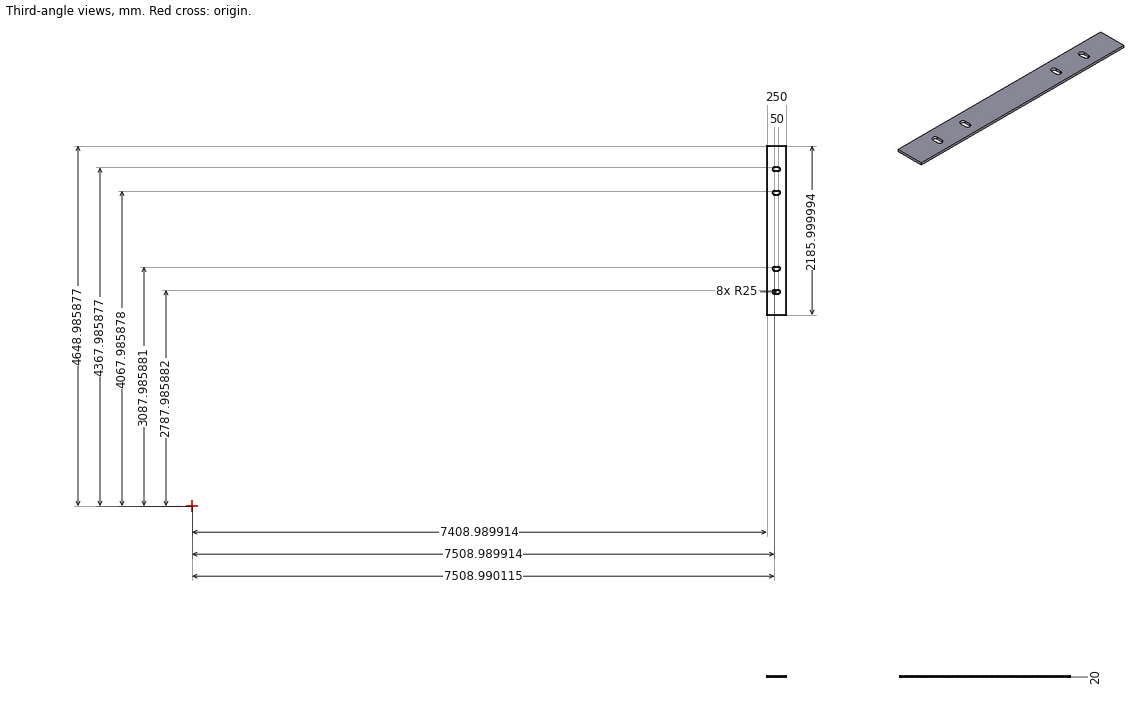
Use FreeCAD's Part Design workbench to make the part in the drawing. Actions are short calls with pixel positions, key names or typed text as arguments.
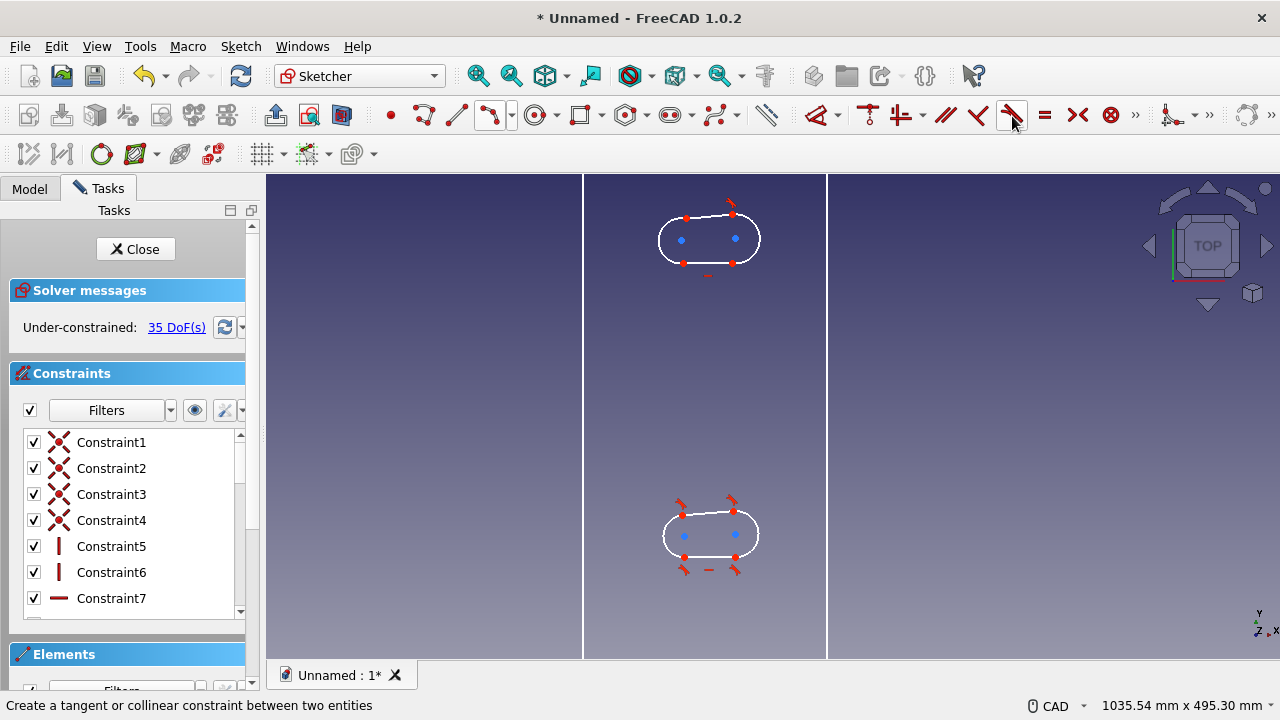
click(700, 218)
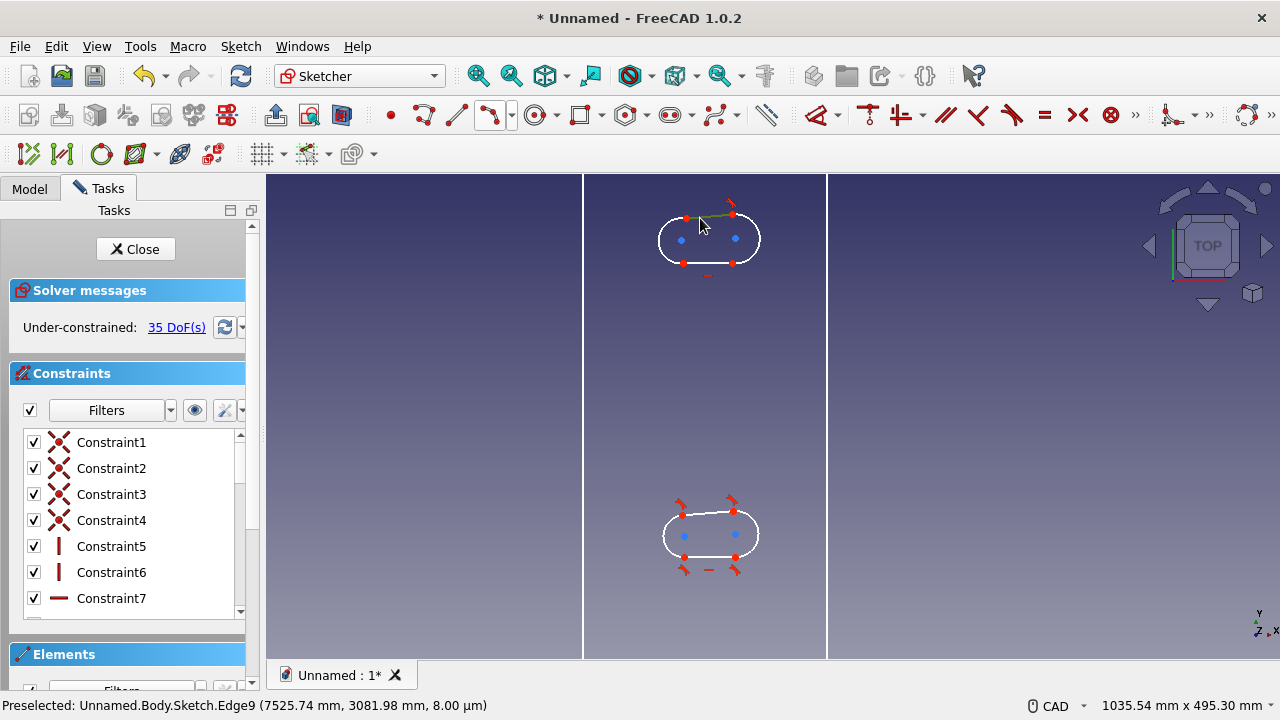
click(665, 225)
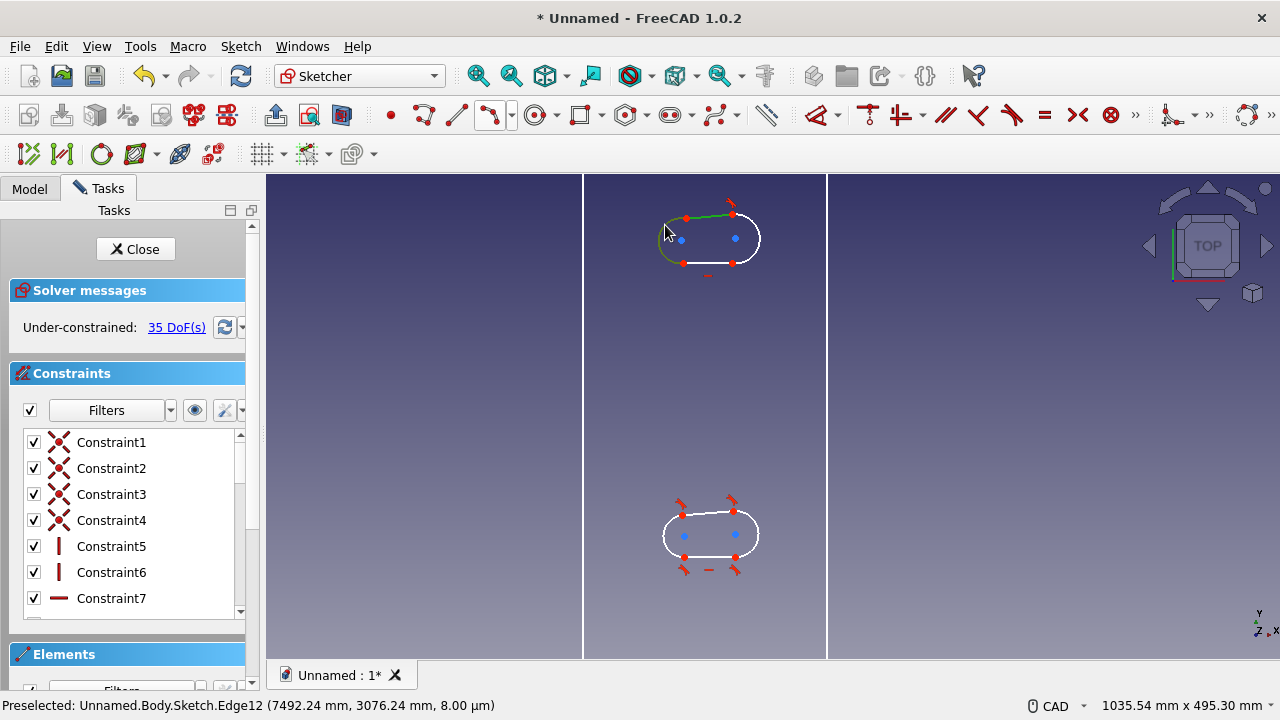
key(t)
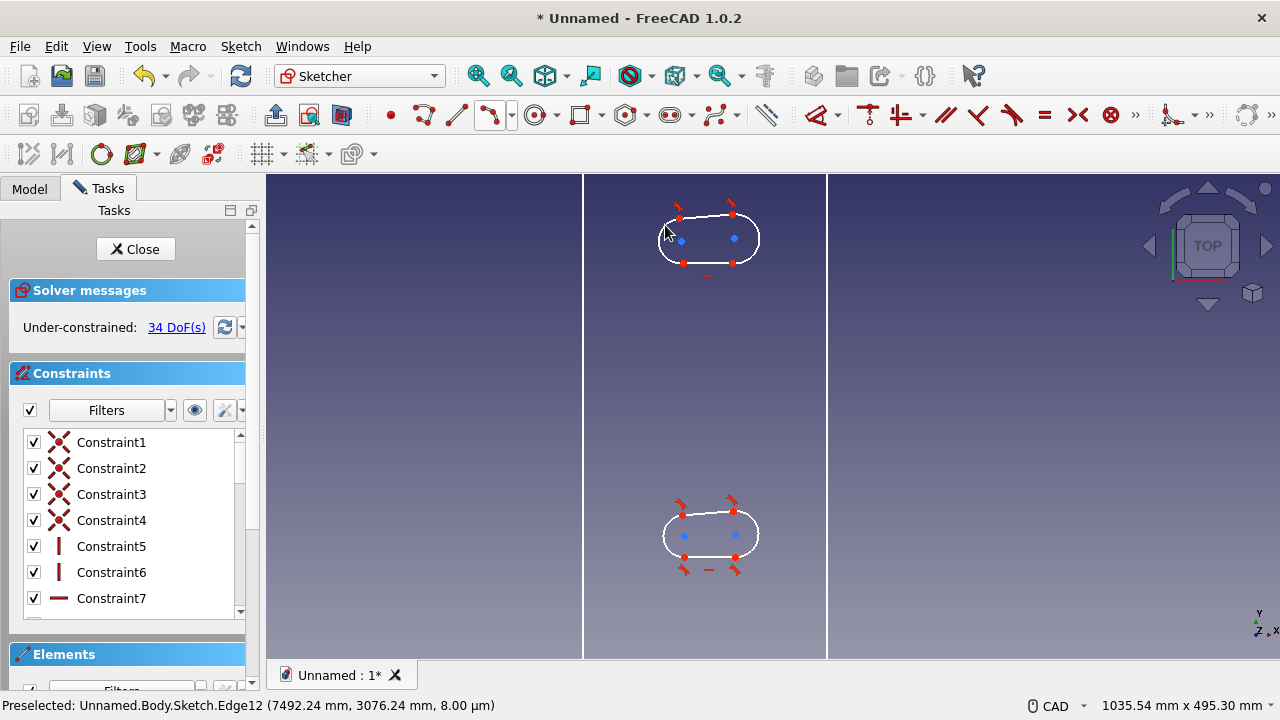
click(718, 263)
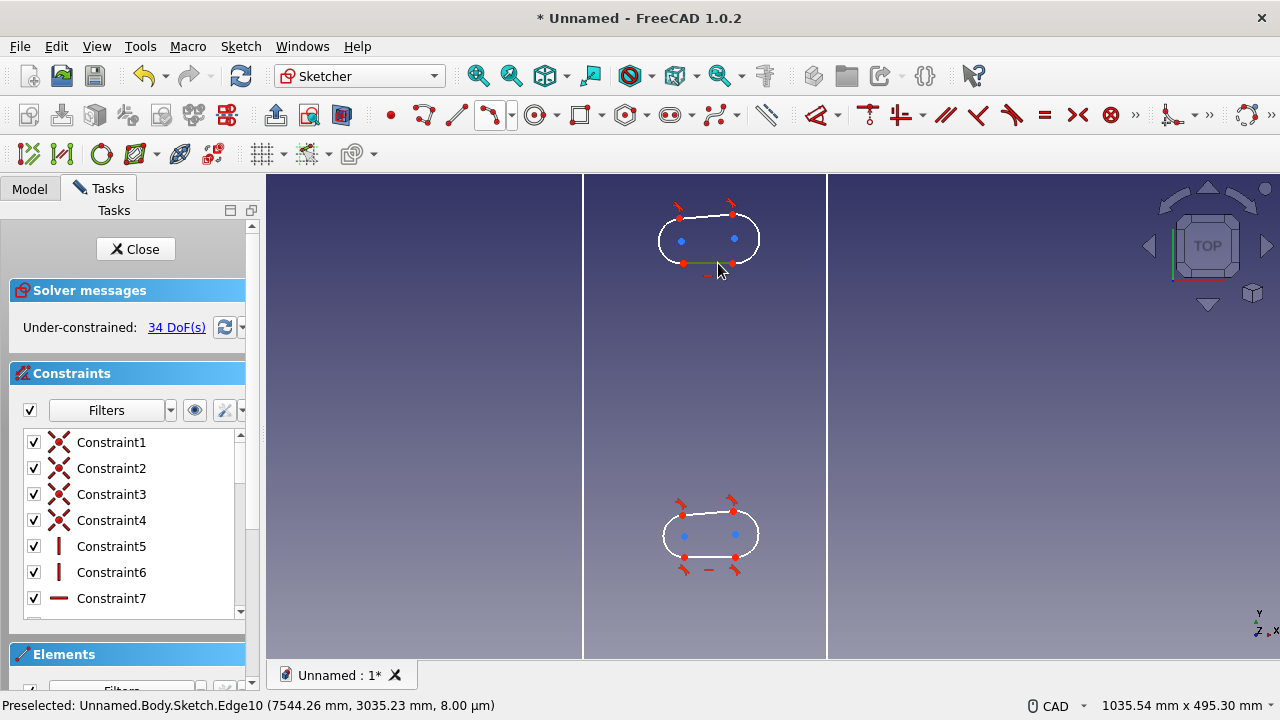
click(754, 254)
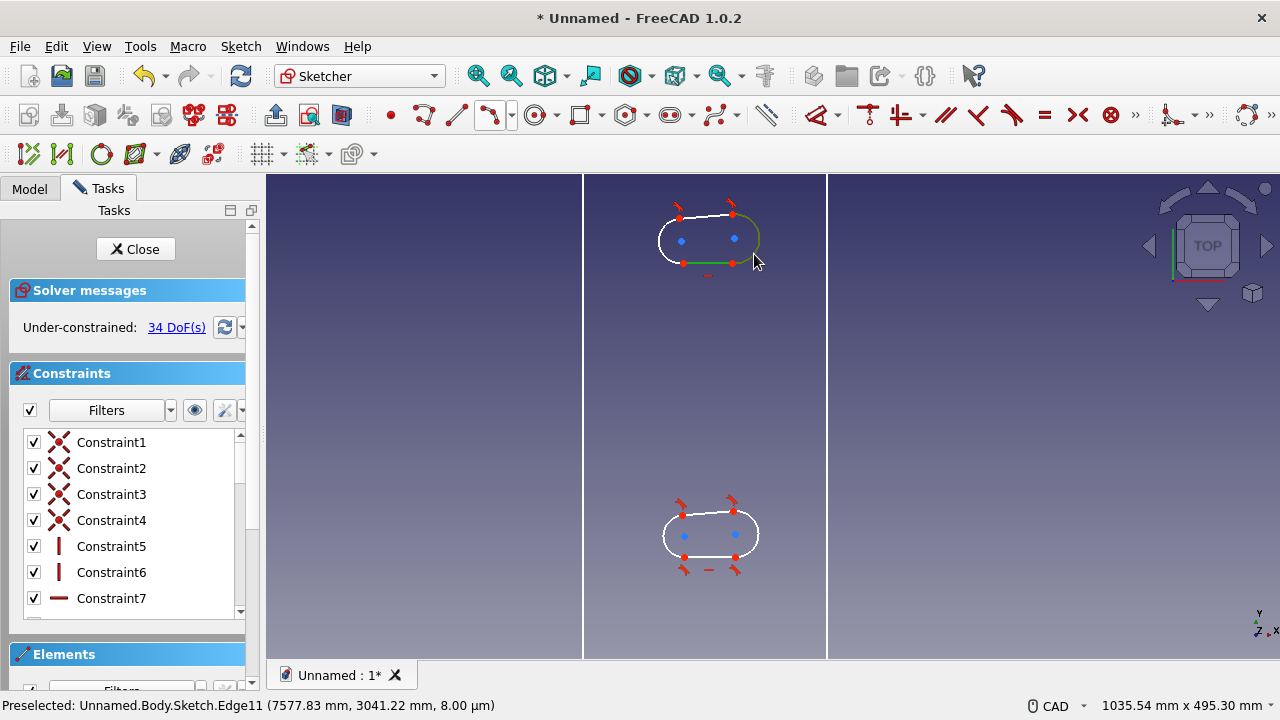
key(t)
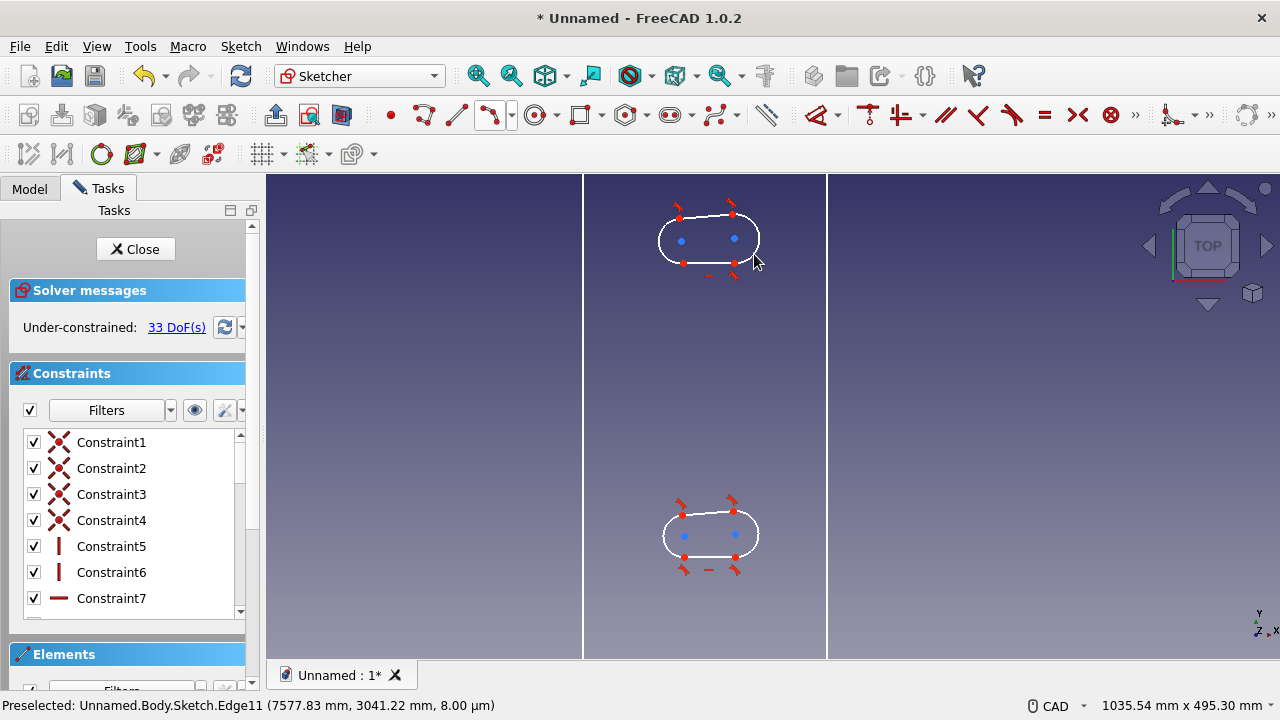
click(720, 263)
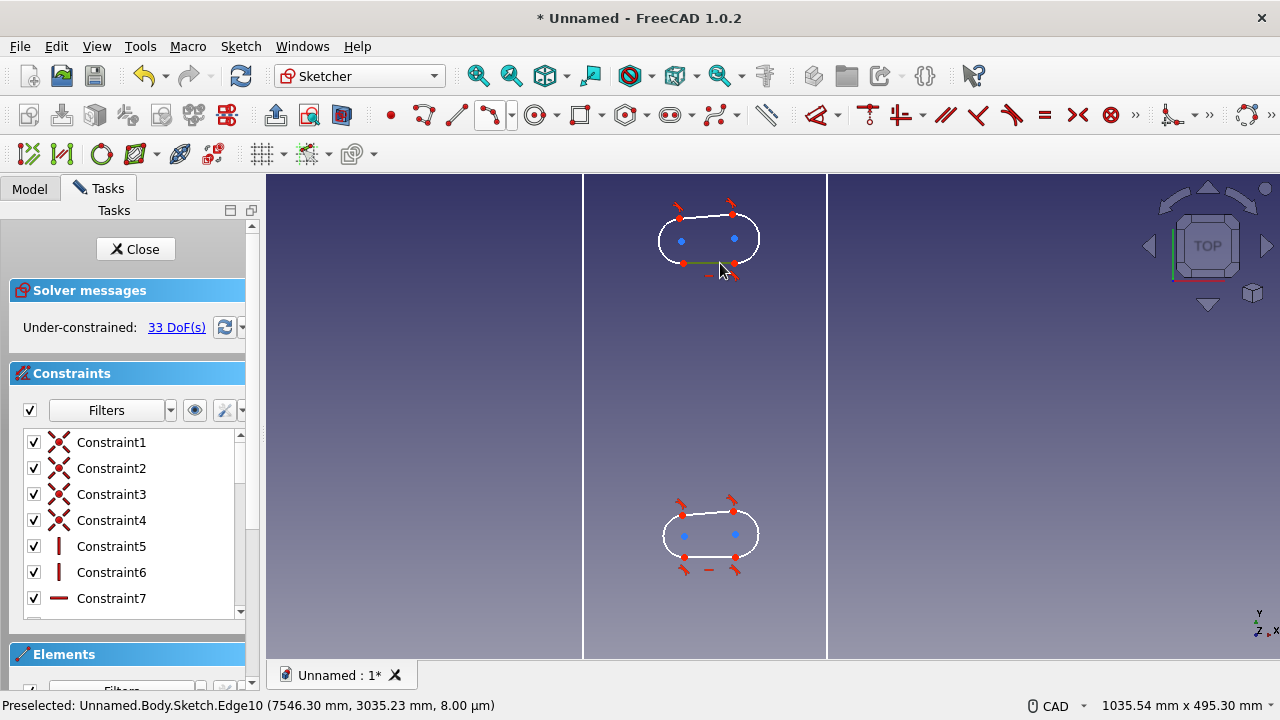
click(662, 230)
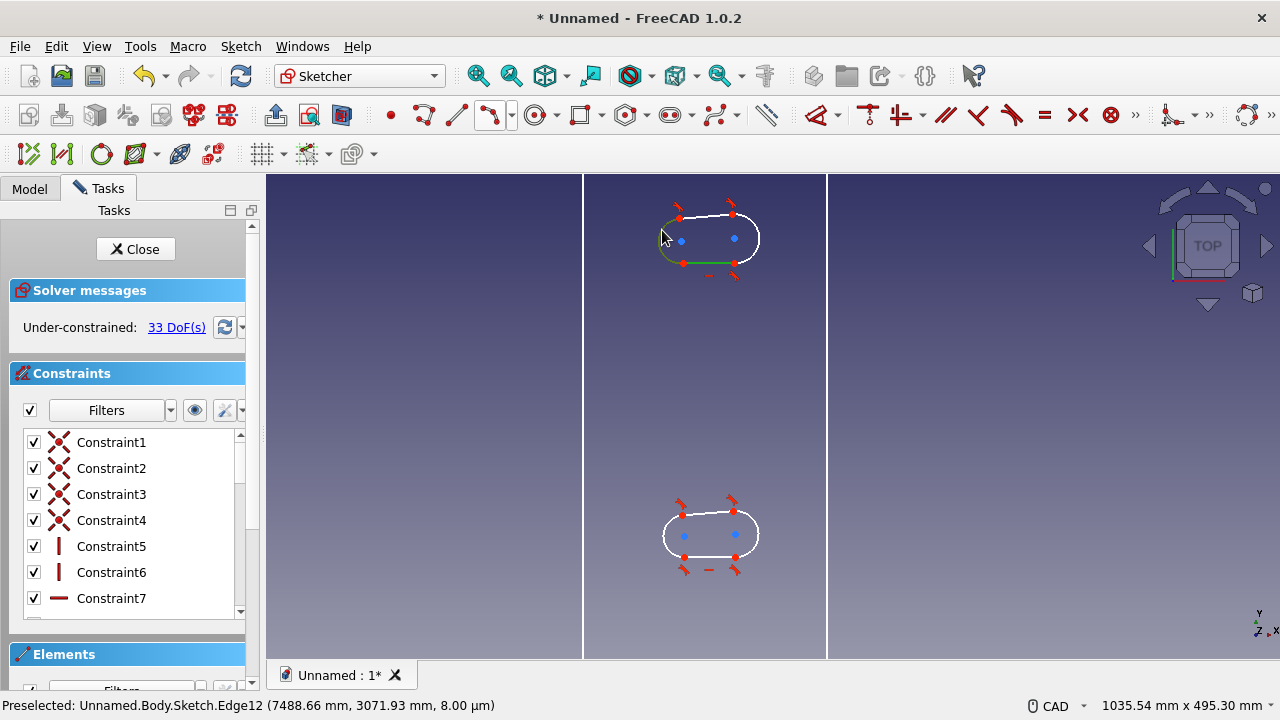
key(t)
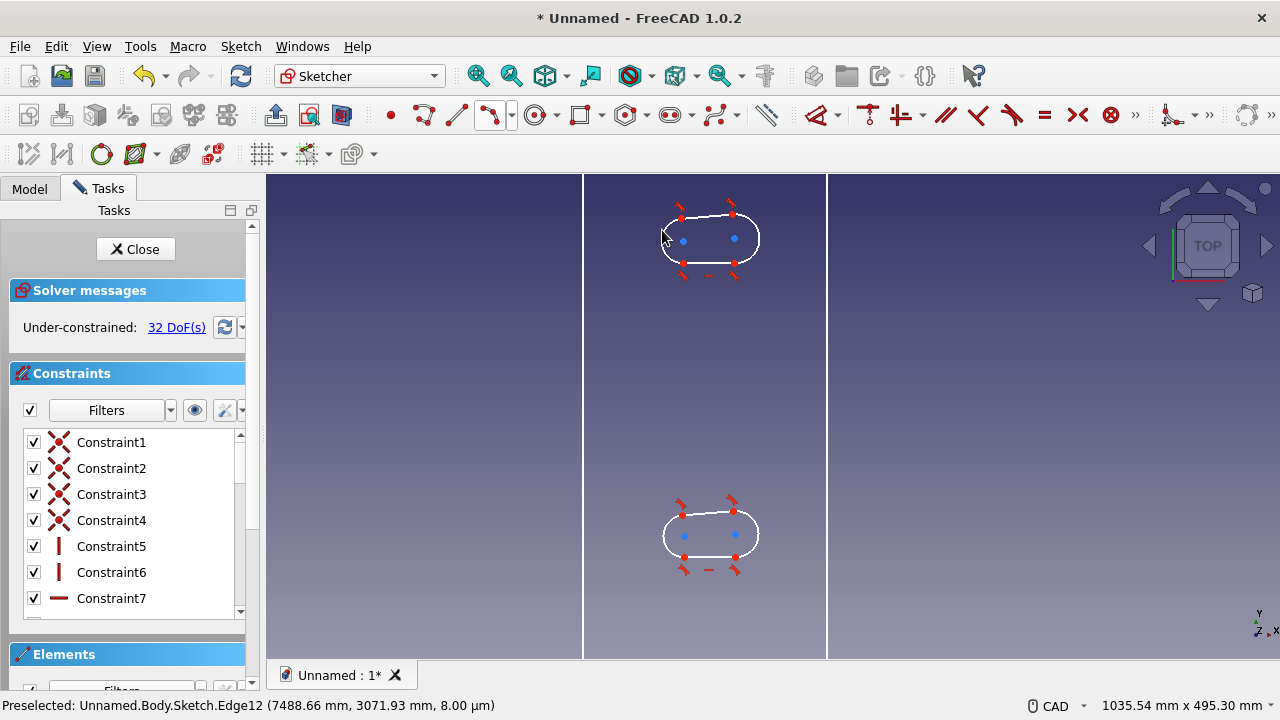
scroll(704, 520, down, 10)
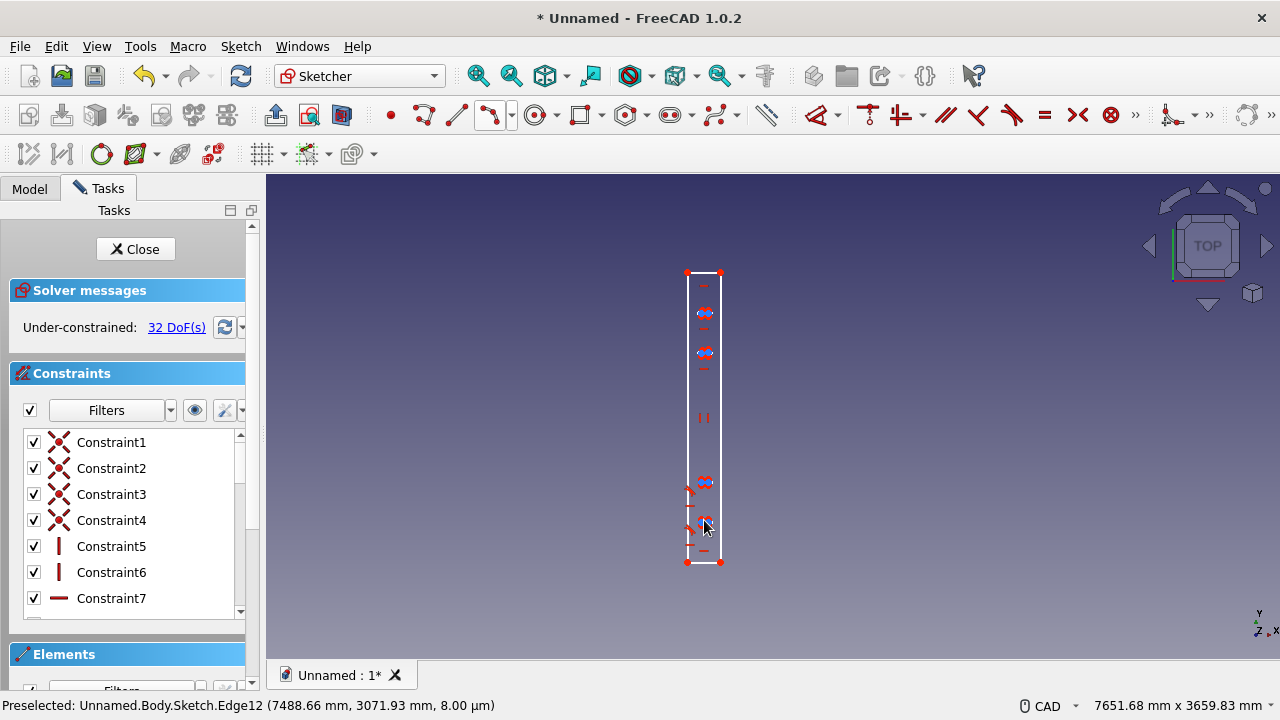
scroll(704, 311, up, 10)